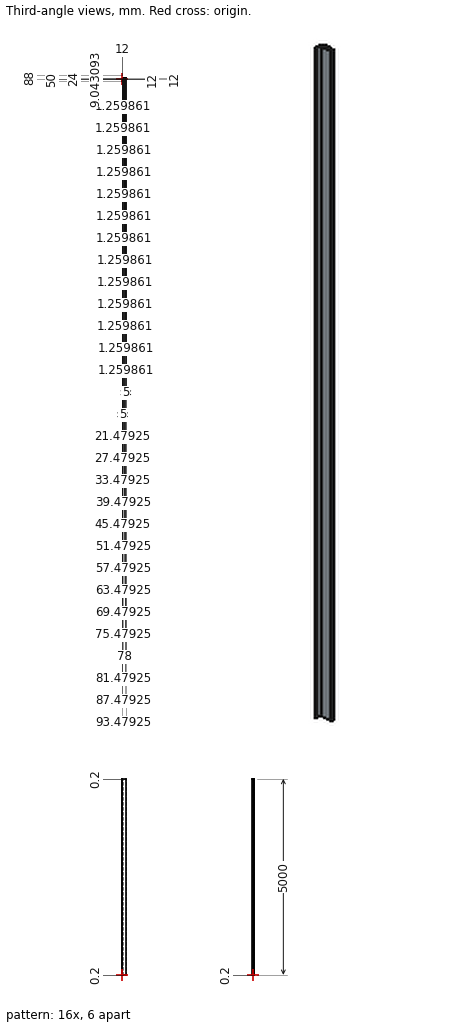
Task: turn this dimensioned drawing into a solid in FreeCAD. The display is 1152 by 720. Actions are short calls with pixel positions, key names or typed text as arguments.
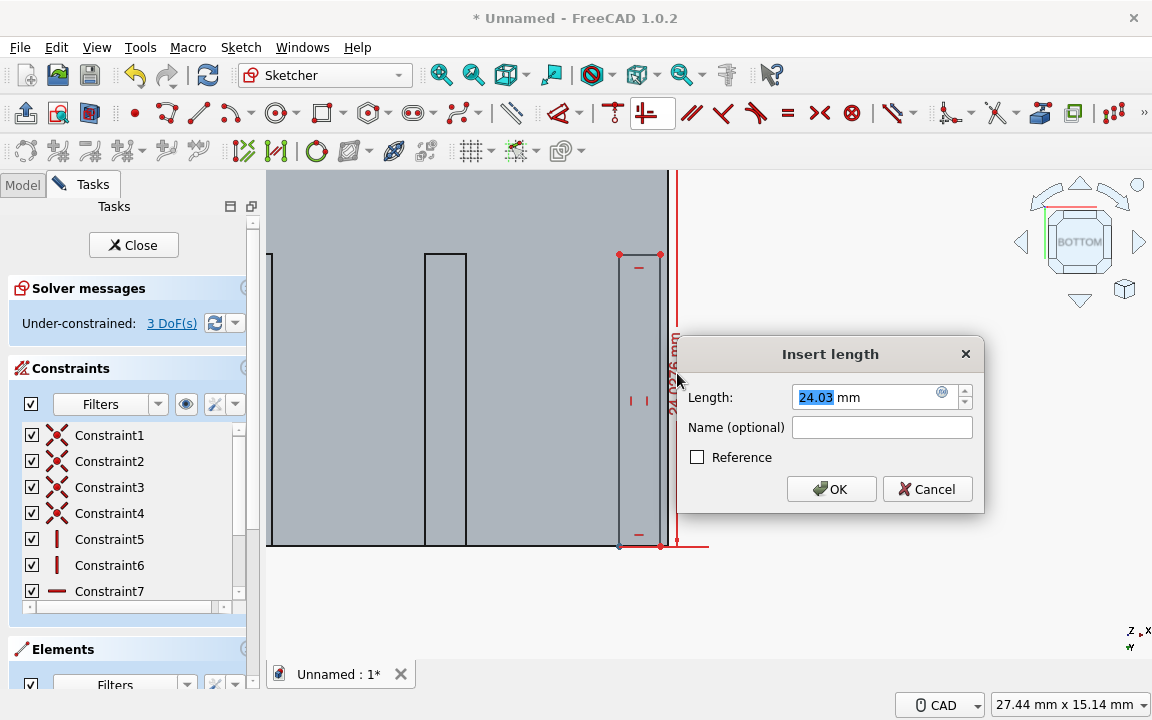
text(24)
key(Return)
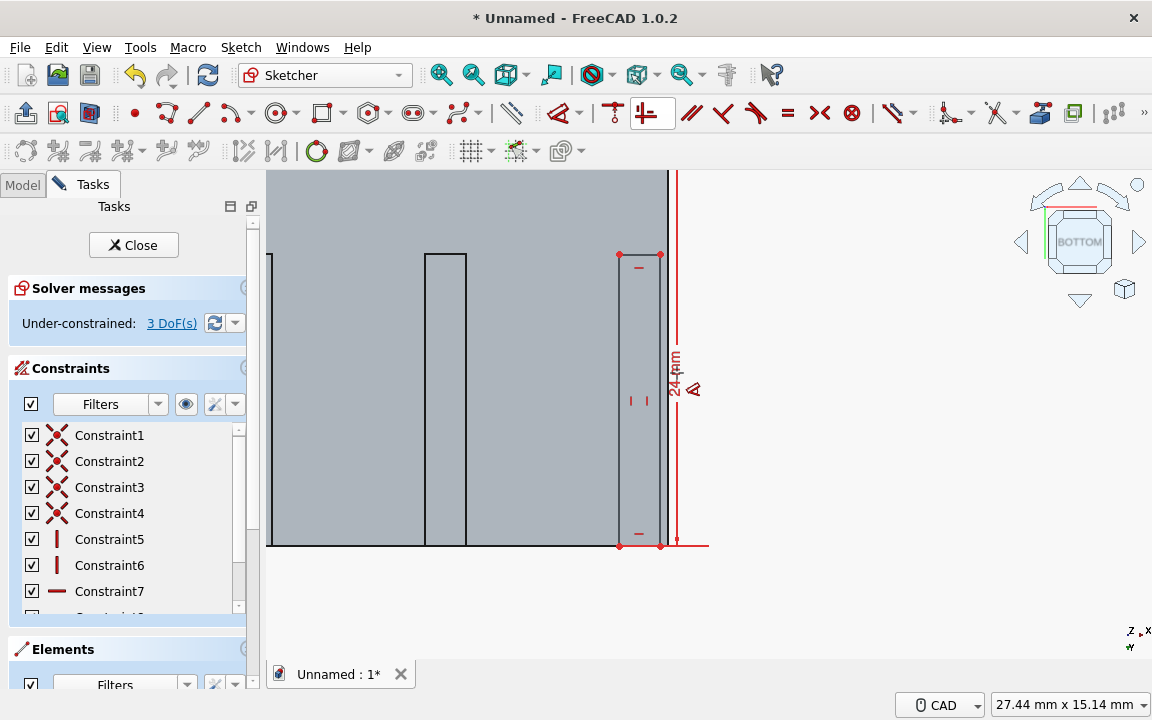
click(619, 342)
click(585, 401)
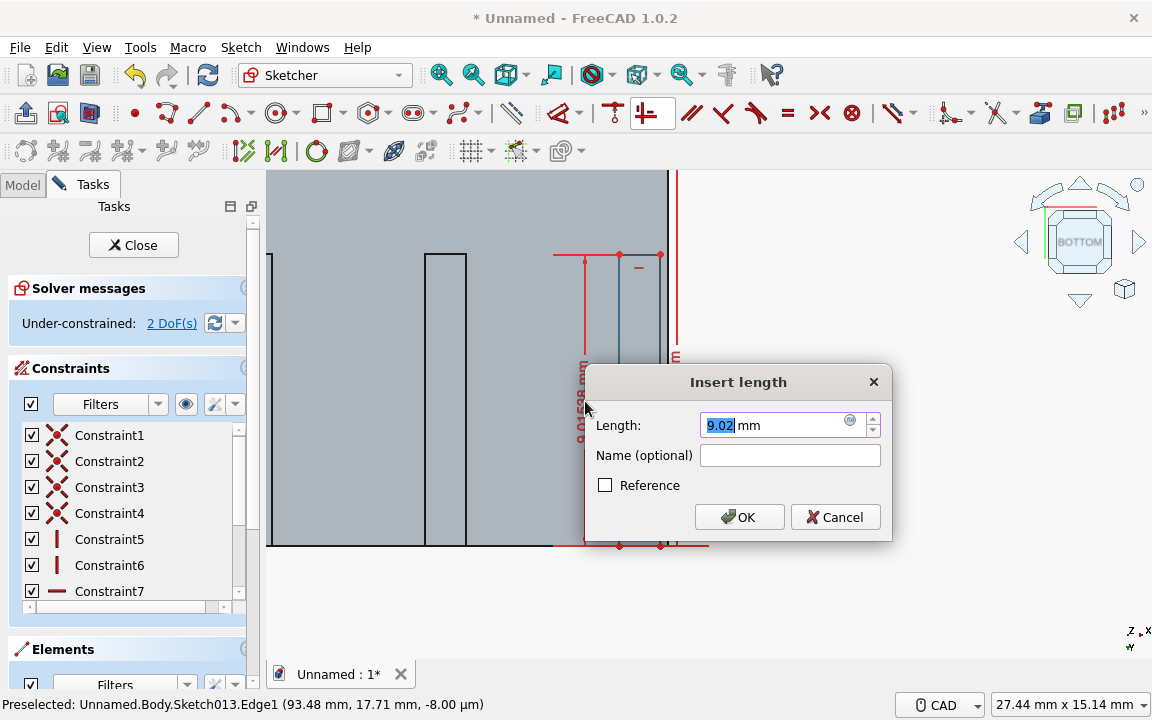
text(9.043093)
key(Return)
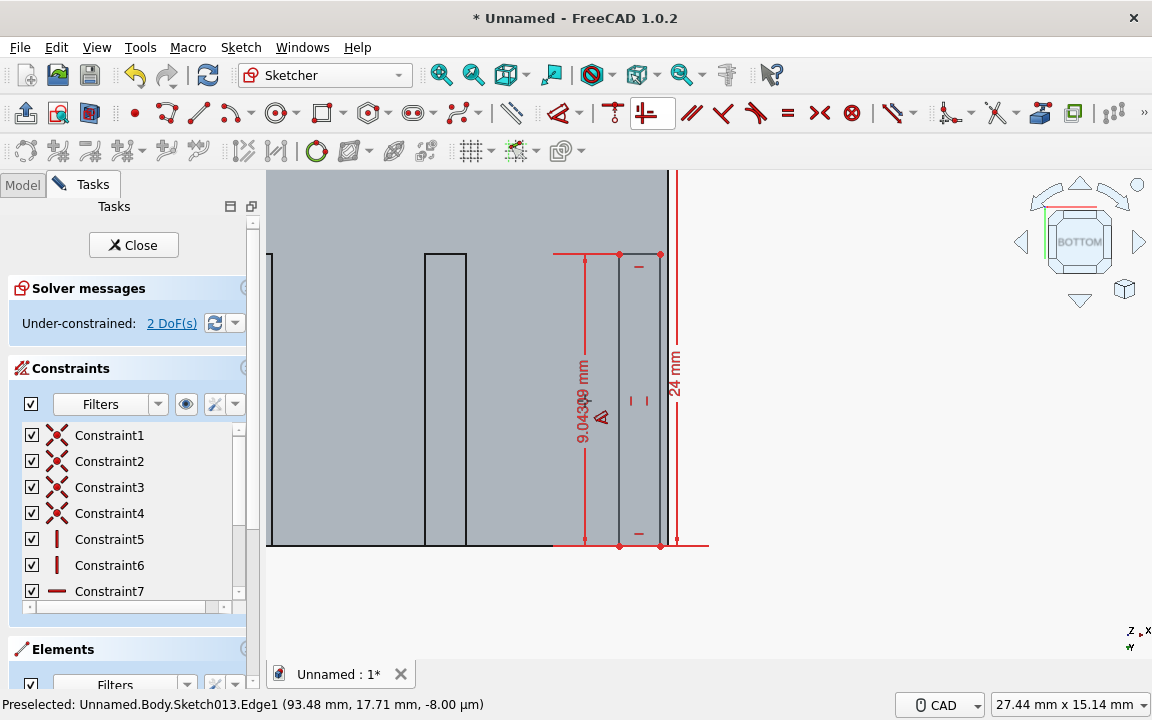
click(631, 546)
click(640, 580)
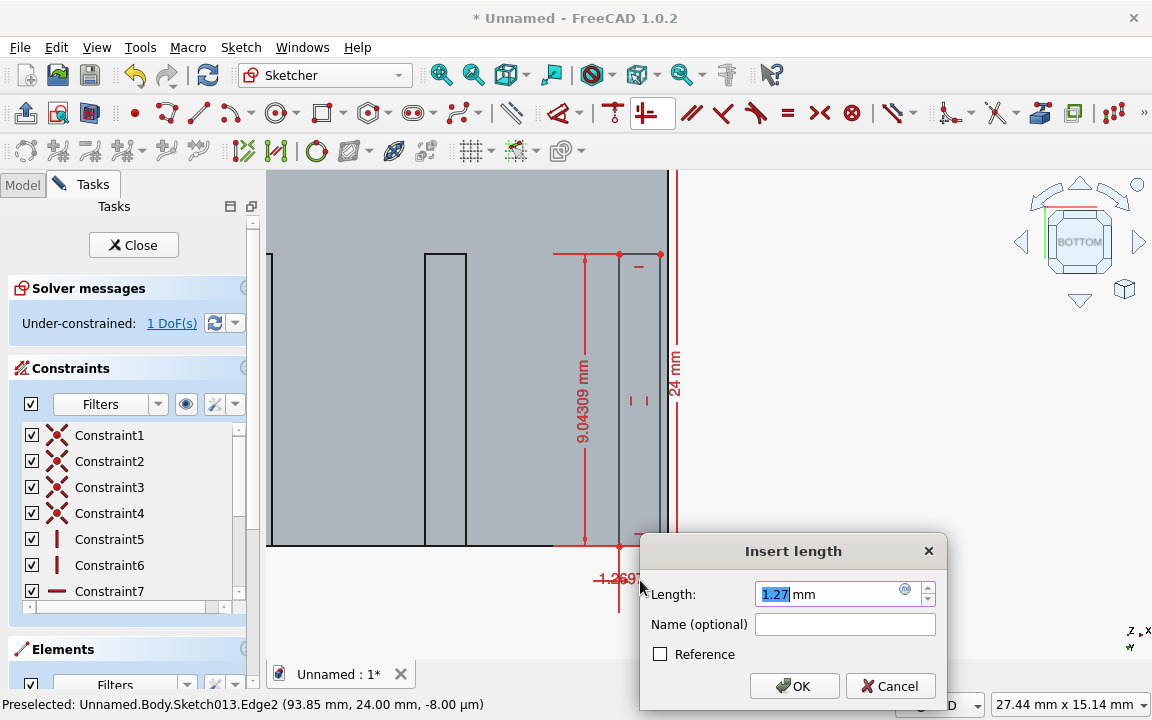
text(1.259861)
key(Return)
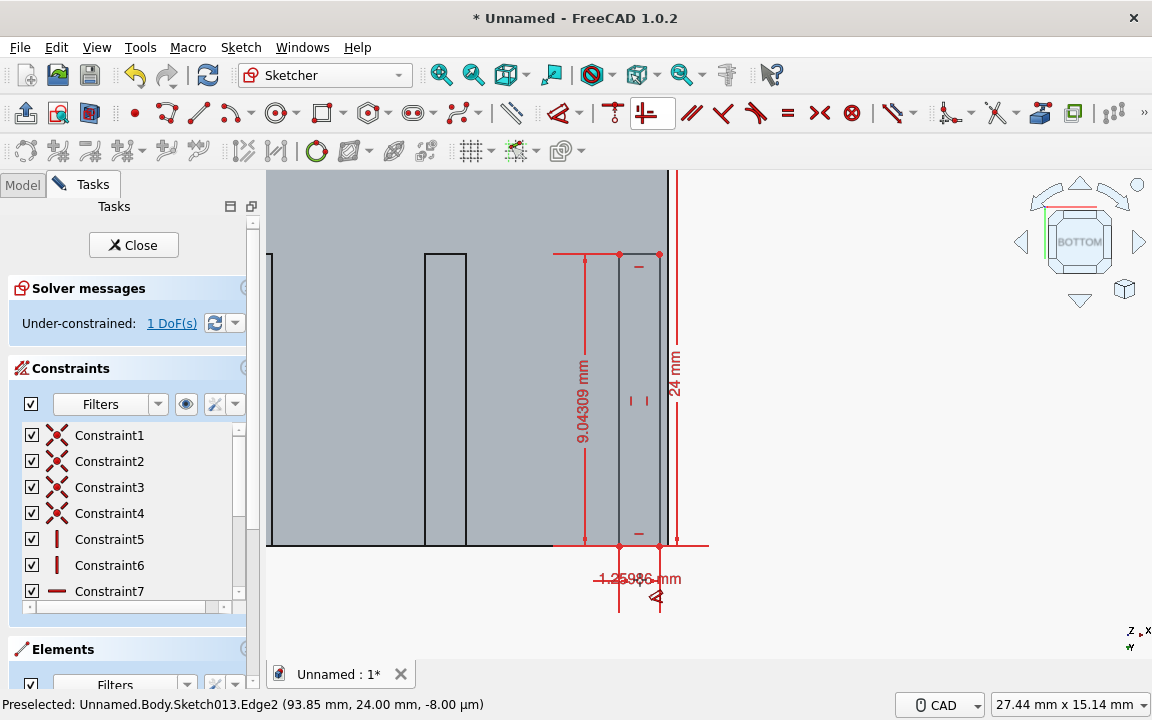
click(619, 254)
click(457, 288)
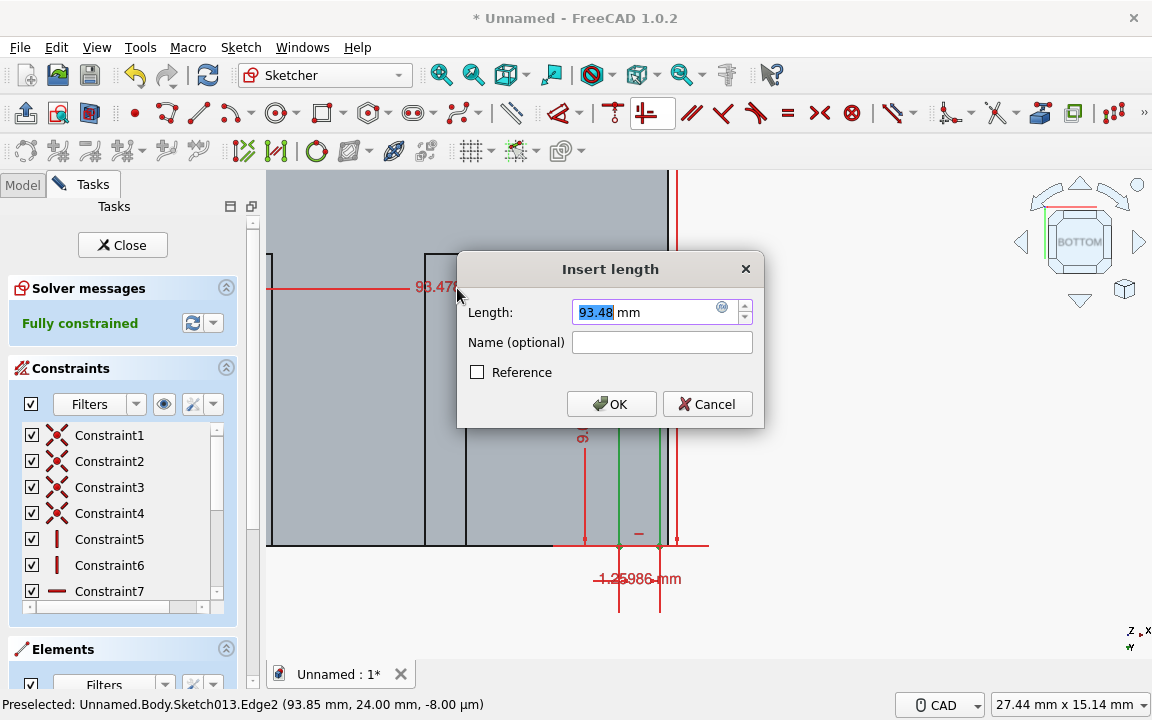
text(93.47925)
key(Return)
key(Escape)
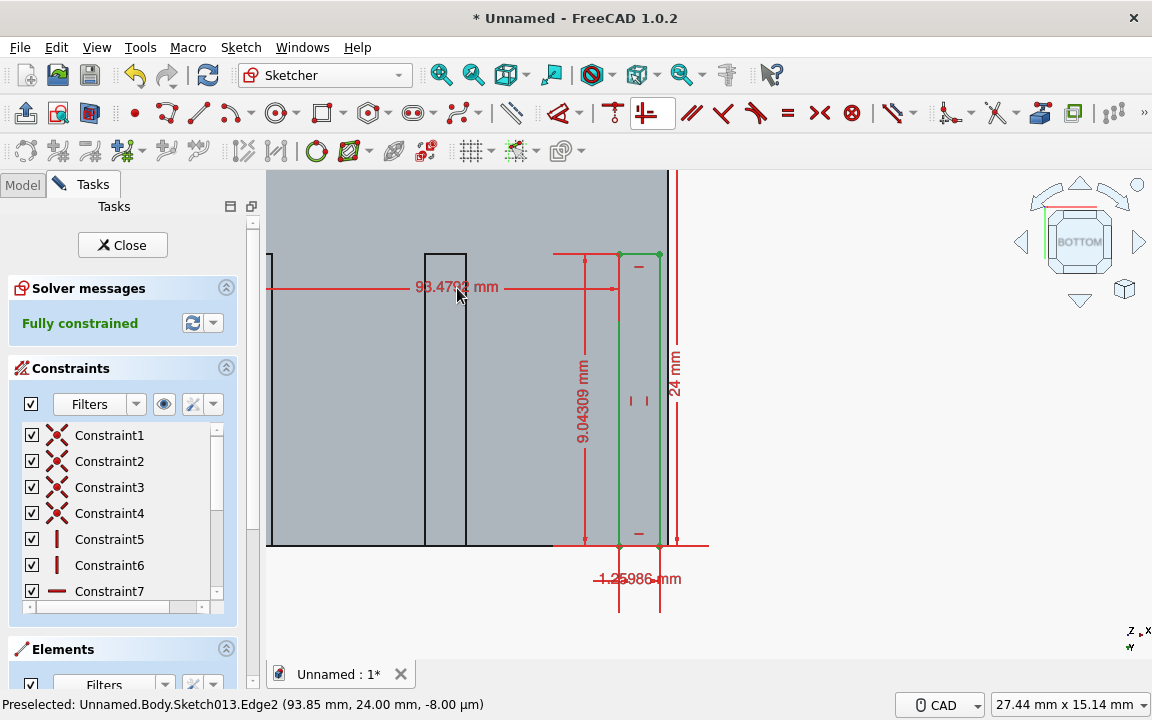
click(123, 245)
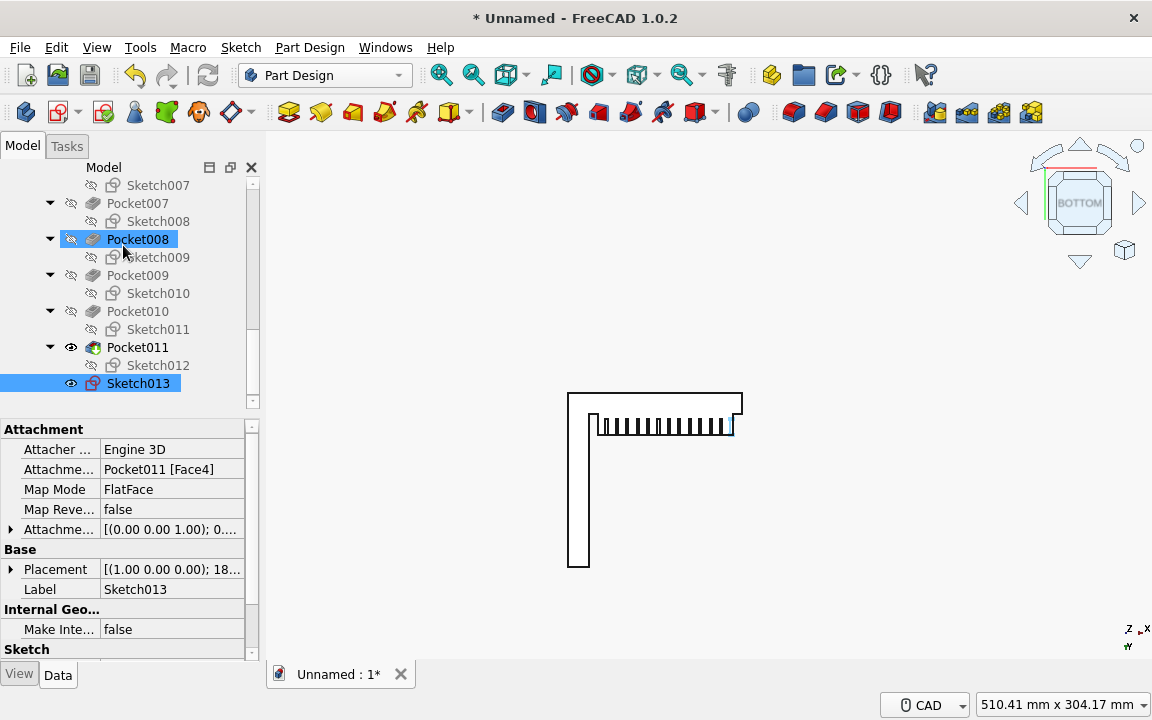
click(504, 112)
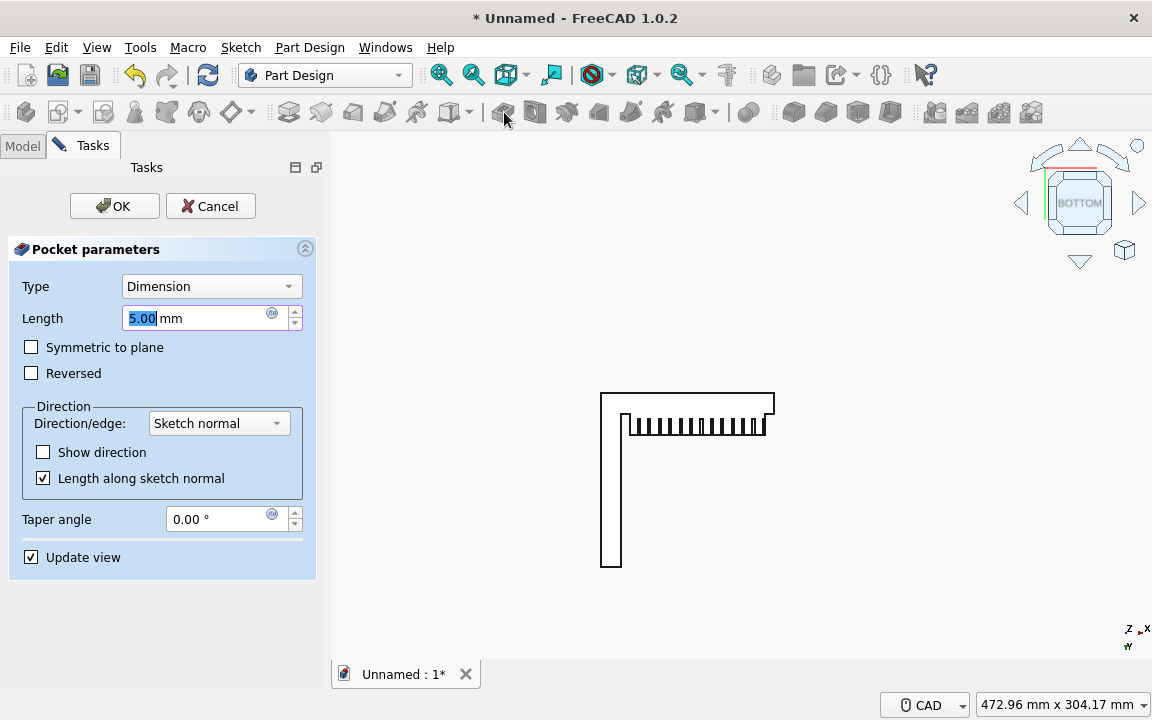
text(0.2)
key(Tab)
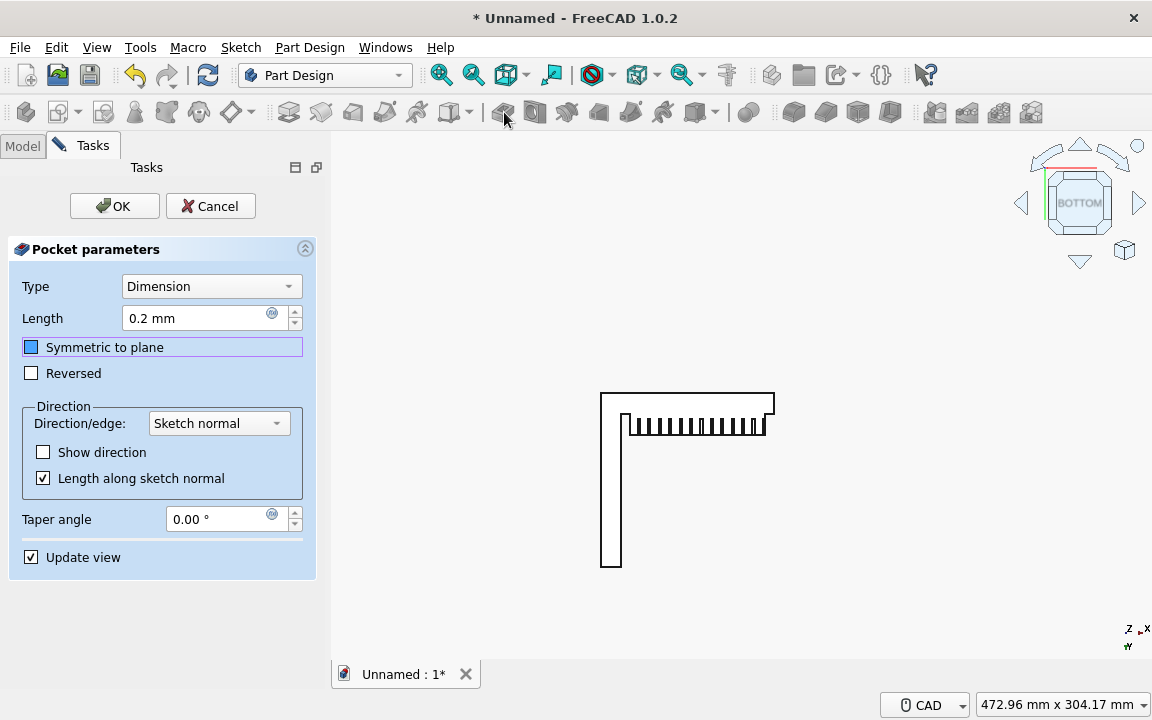
click(115, 206)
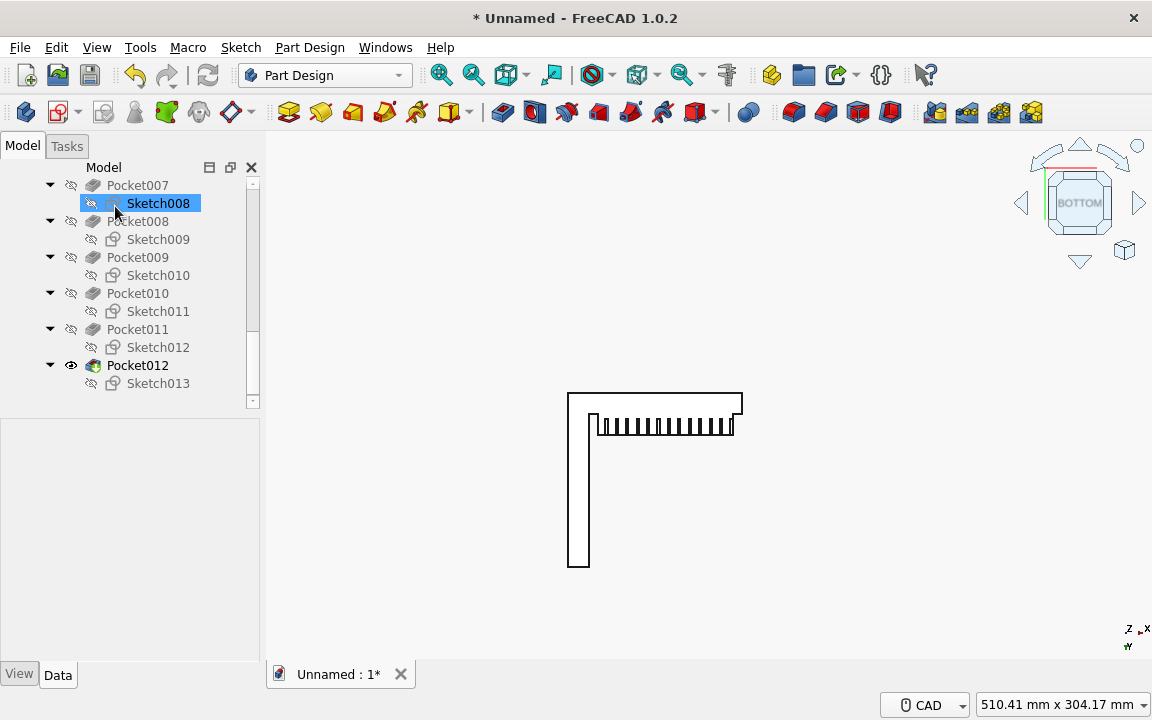
click(442, 76)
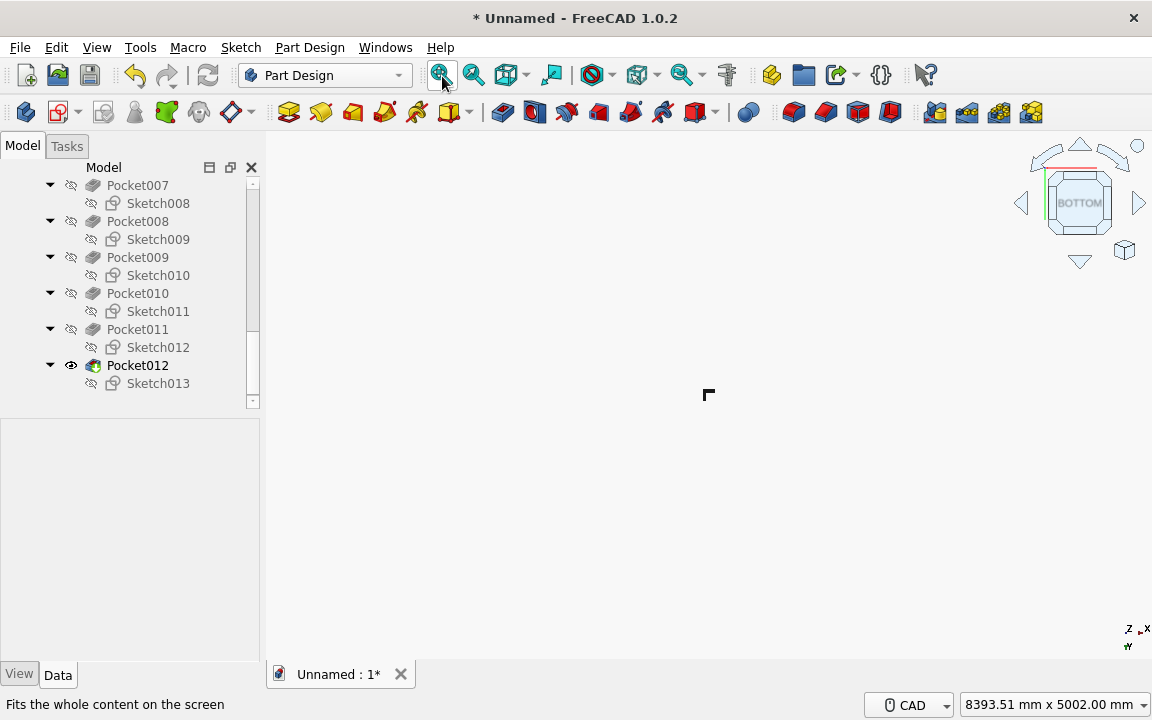
key(0)